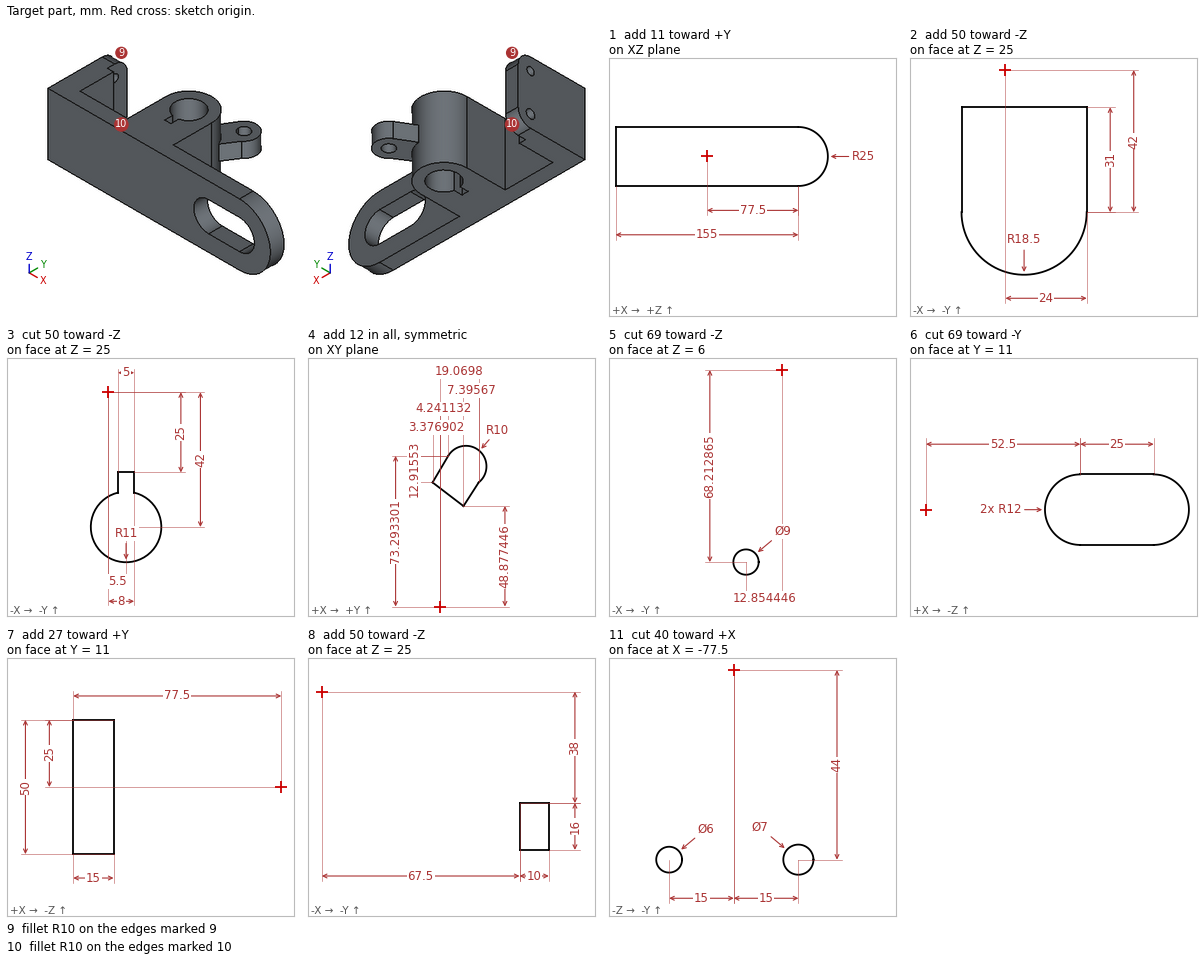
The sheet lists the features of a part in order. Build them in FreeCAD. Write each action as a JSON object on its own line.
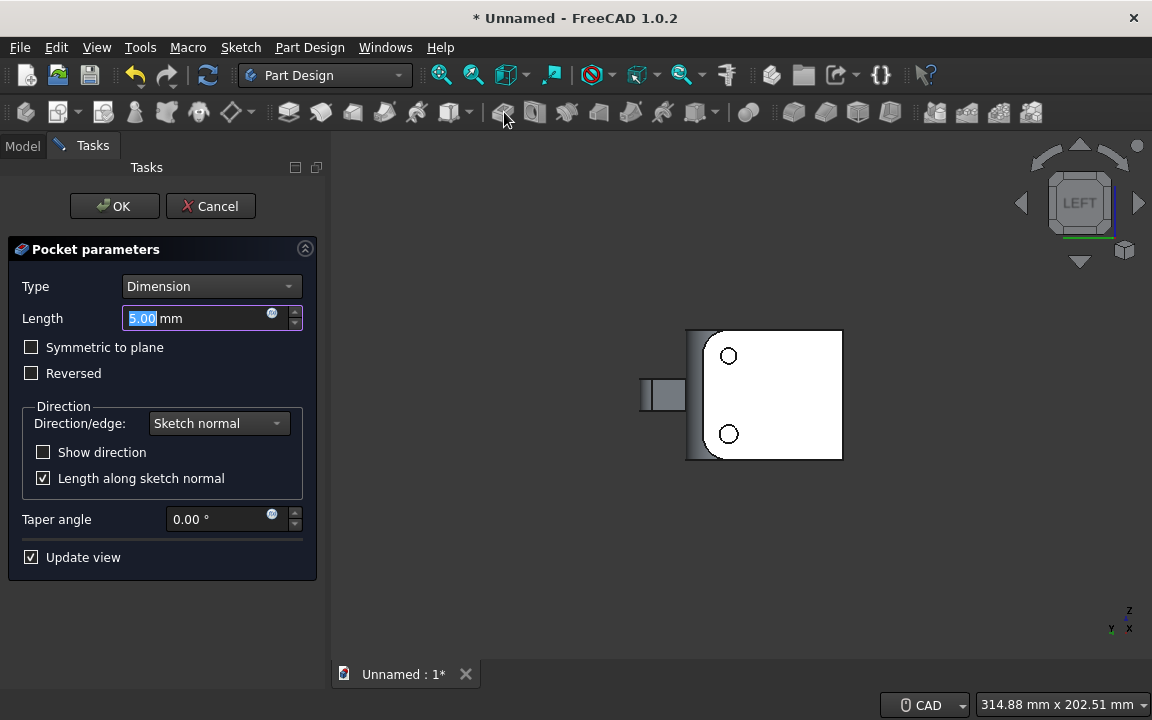
{"action": "type", "text": "40"}
{"action": "key", "text": "Tab"}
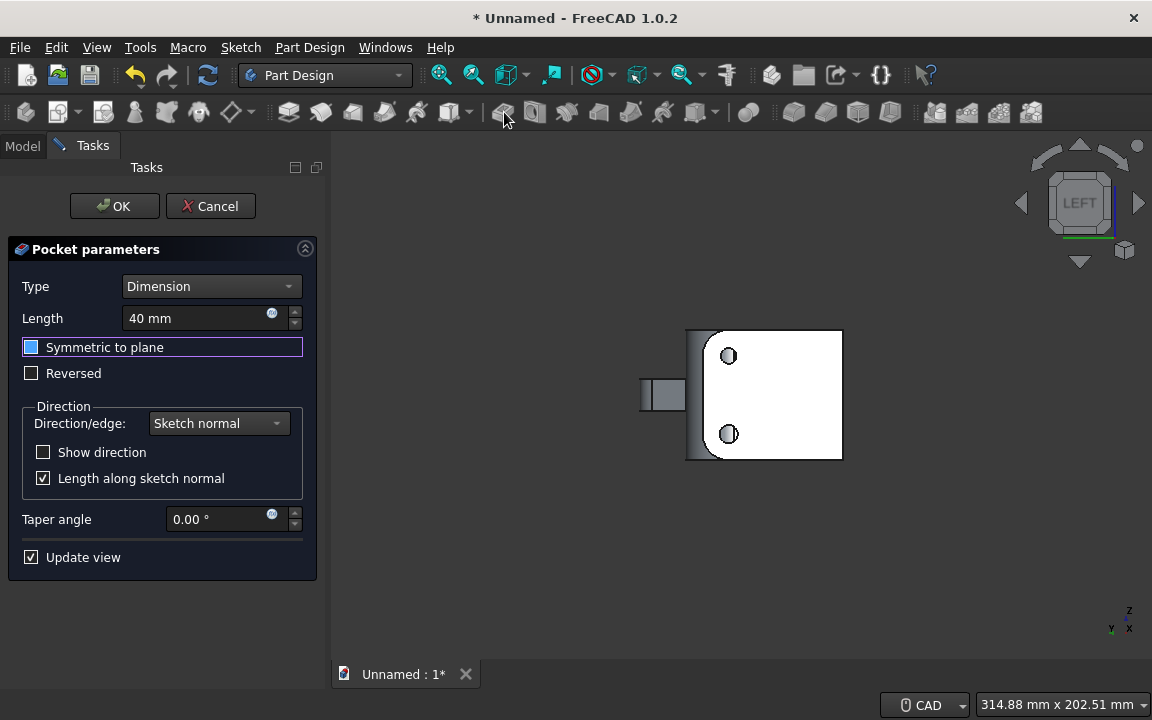
{"action": "left_click", "coordinate": [115, 206]}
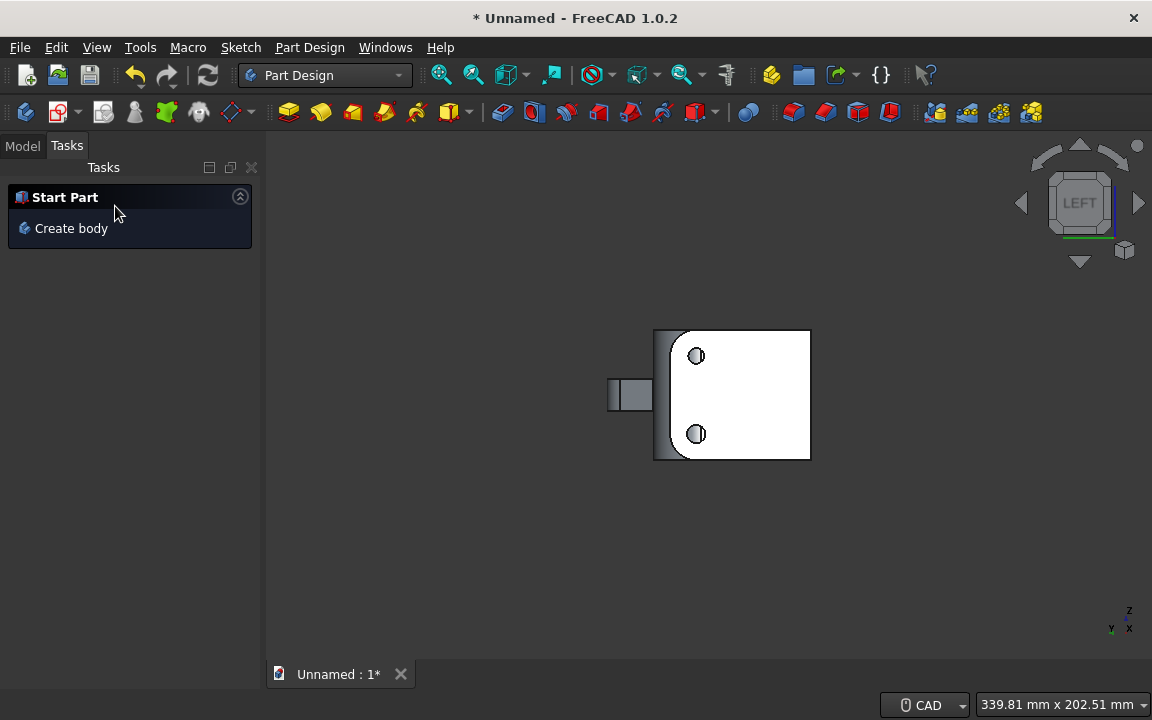
{"action": "key", "text": "0"}